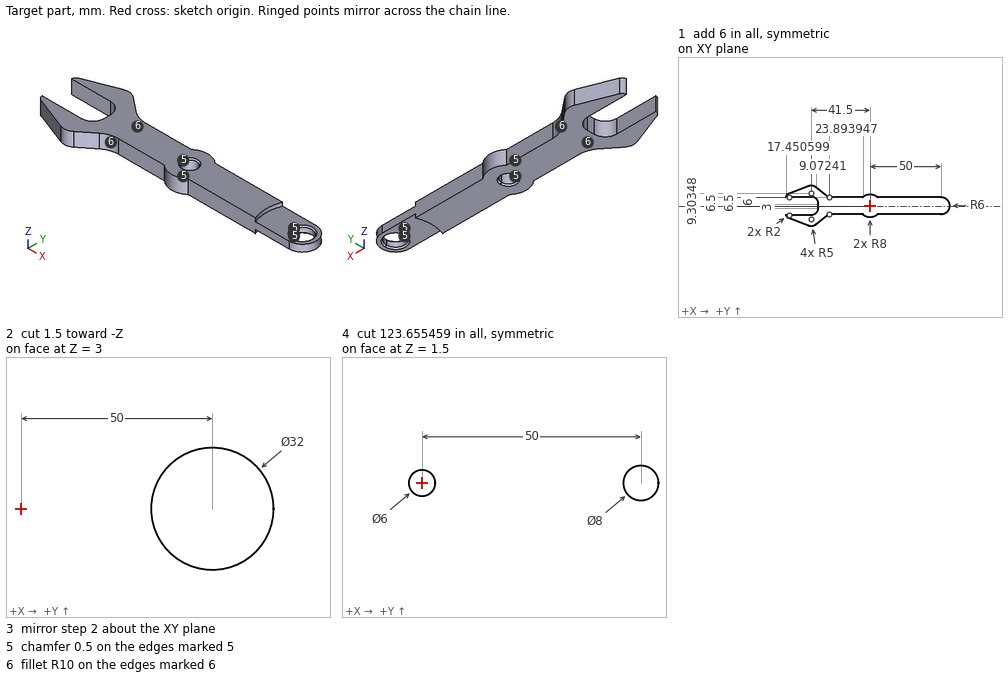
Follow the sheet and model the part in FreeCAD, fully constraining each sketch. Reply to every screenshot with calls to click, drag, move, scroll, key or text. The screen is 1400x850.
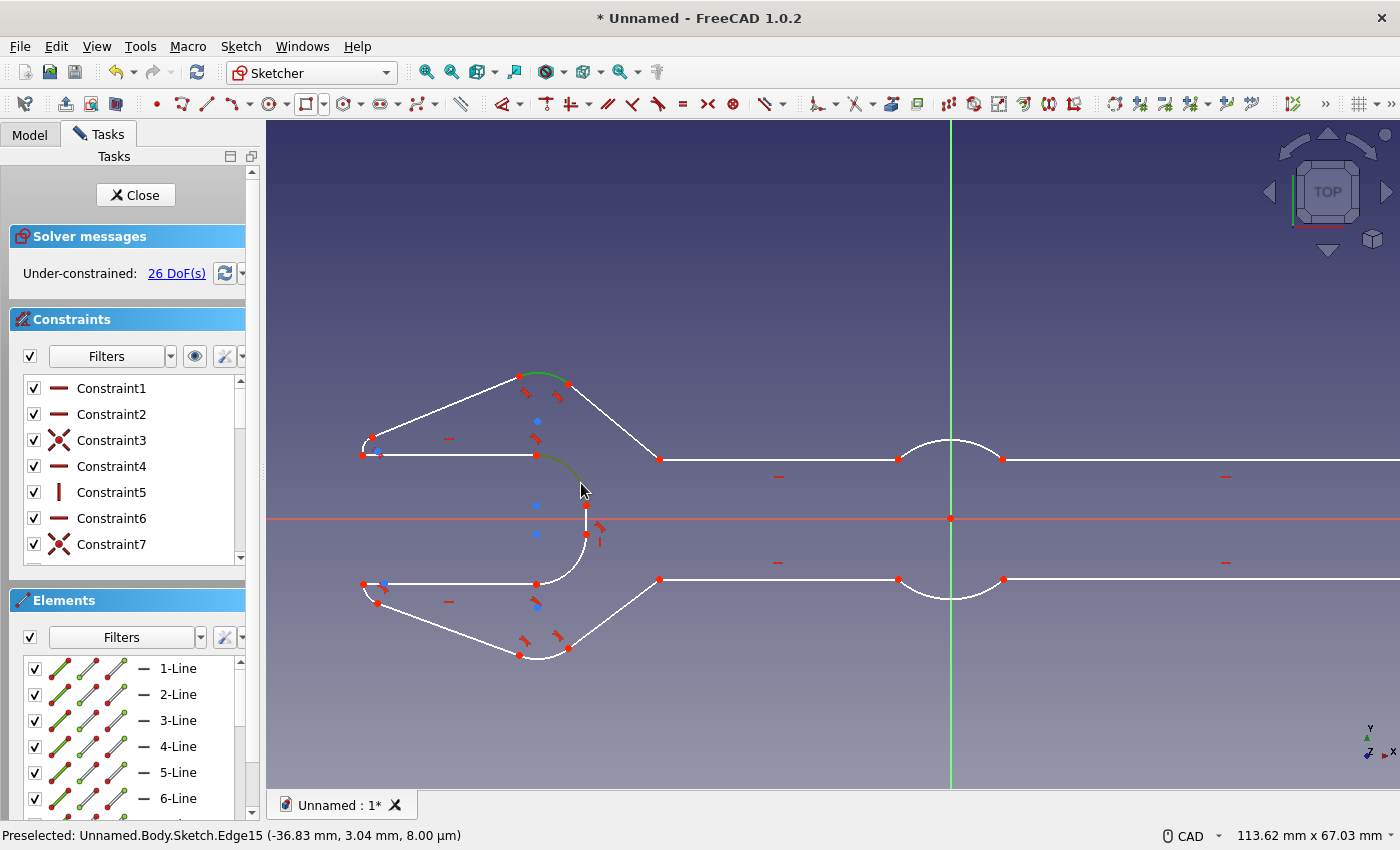
click(559, 579)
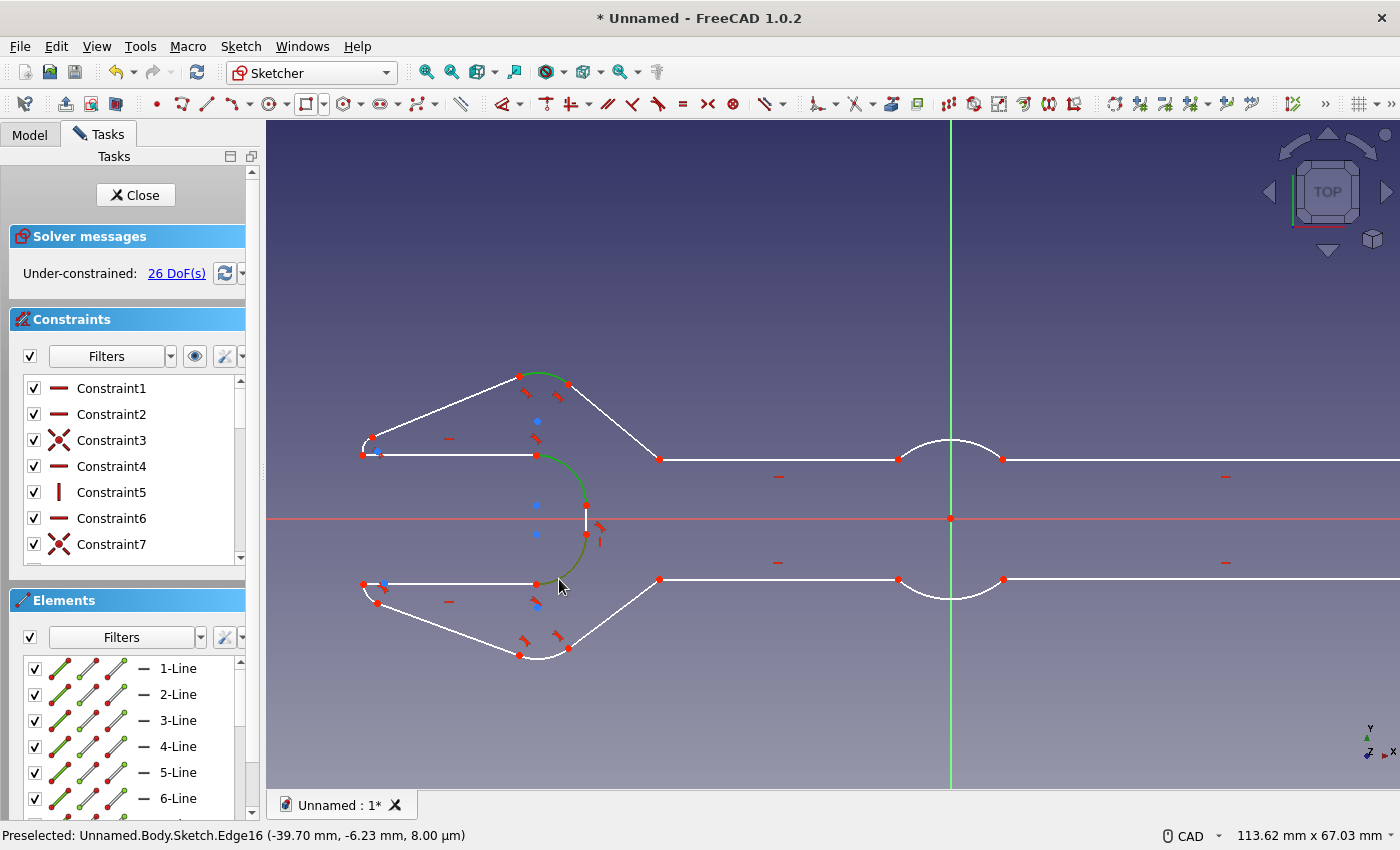
click(535, 659)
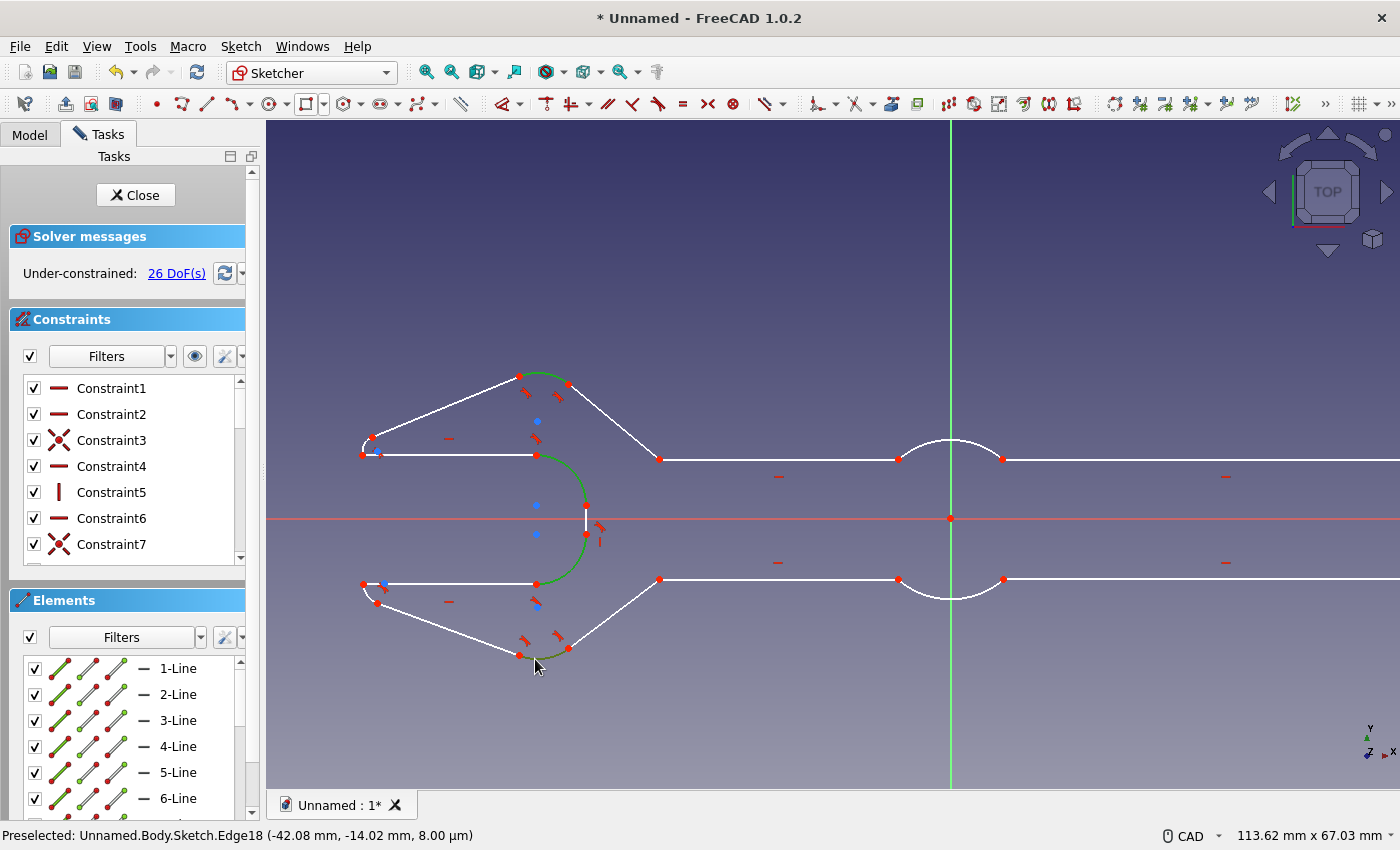
click(683, 104)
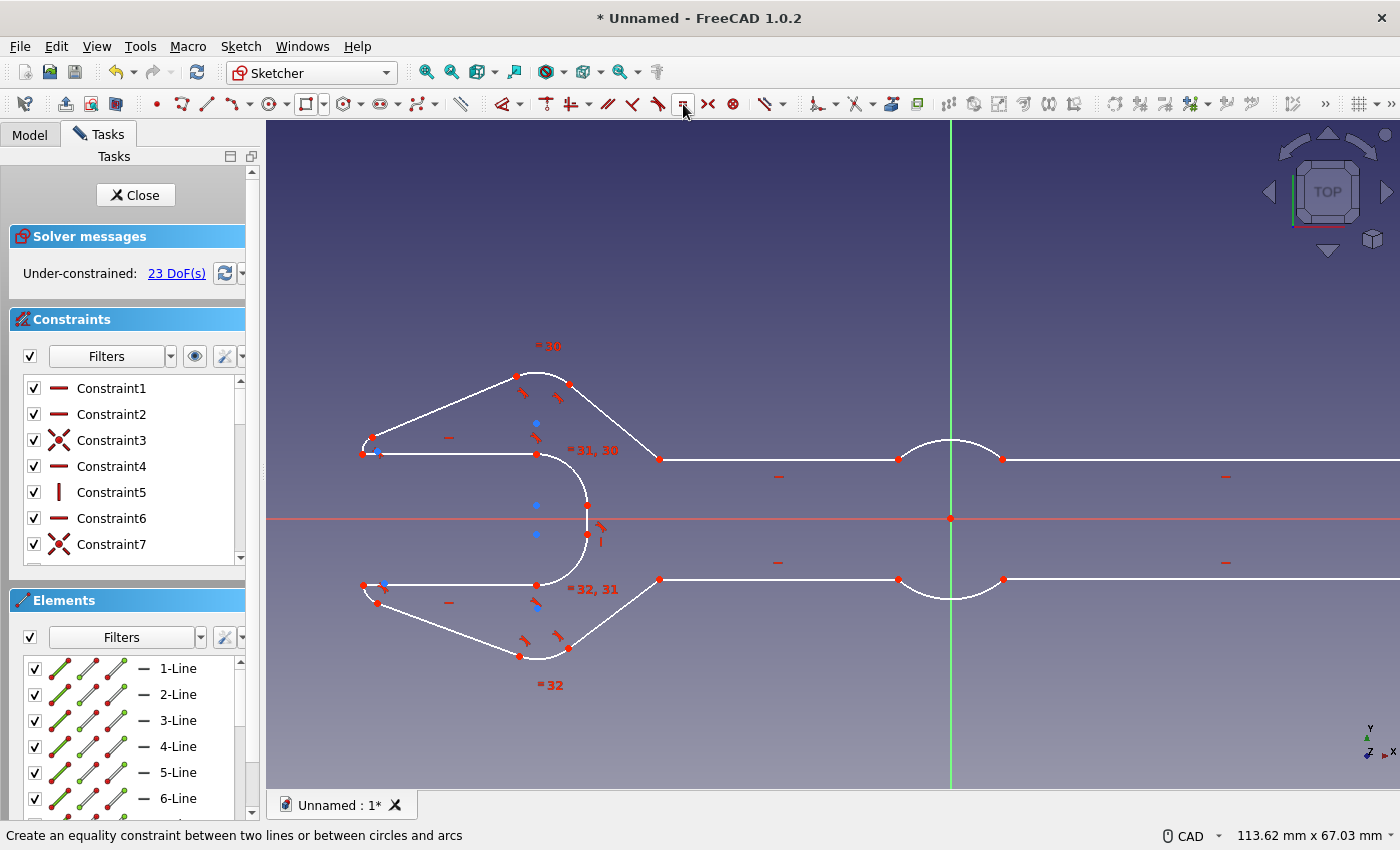
scroll(365, 444, up, 2)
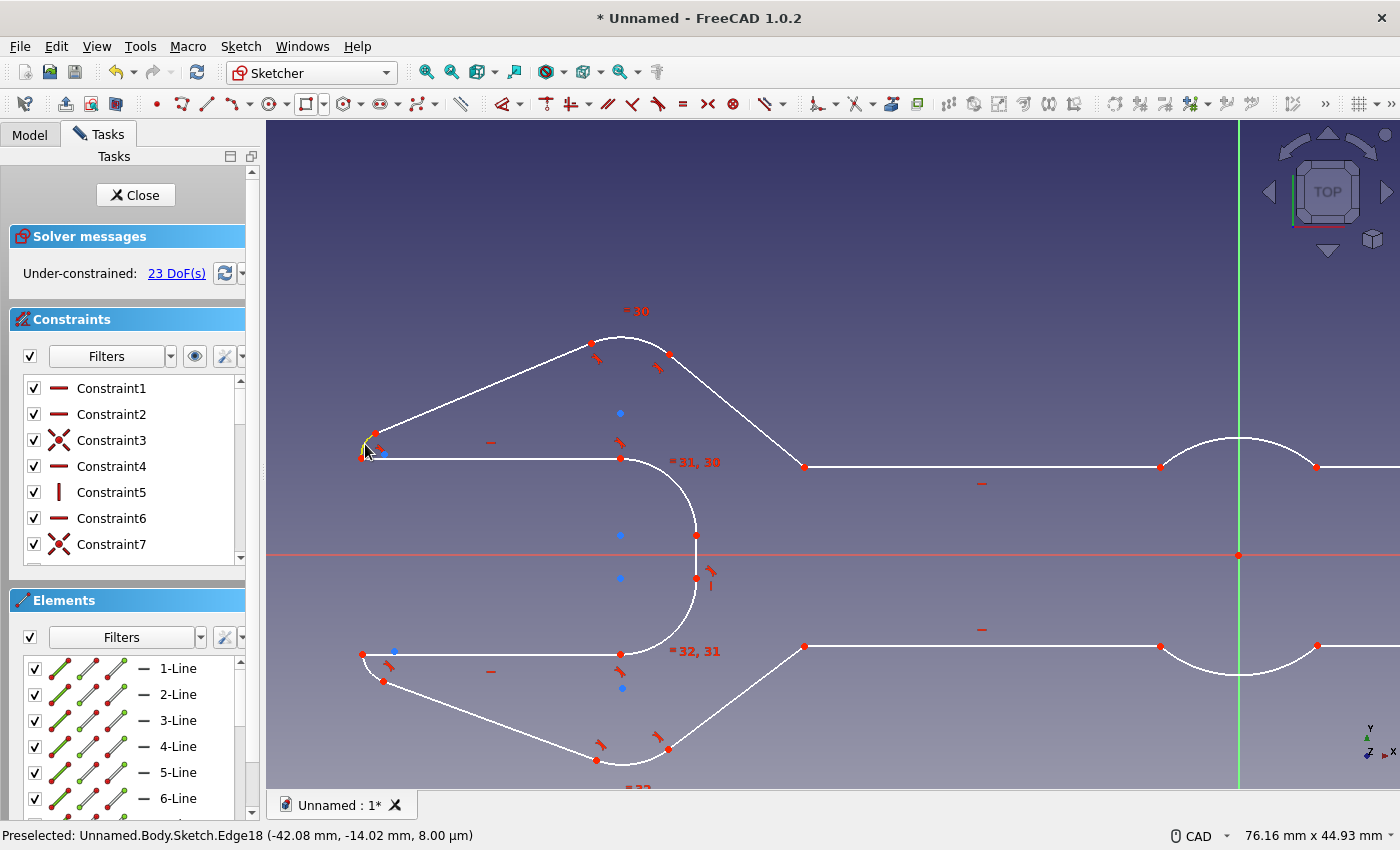
click(364, 444)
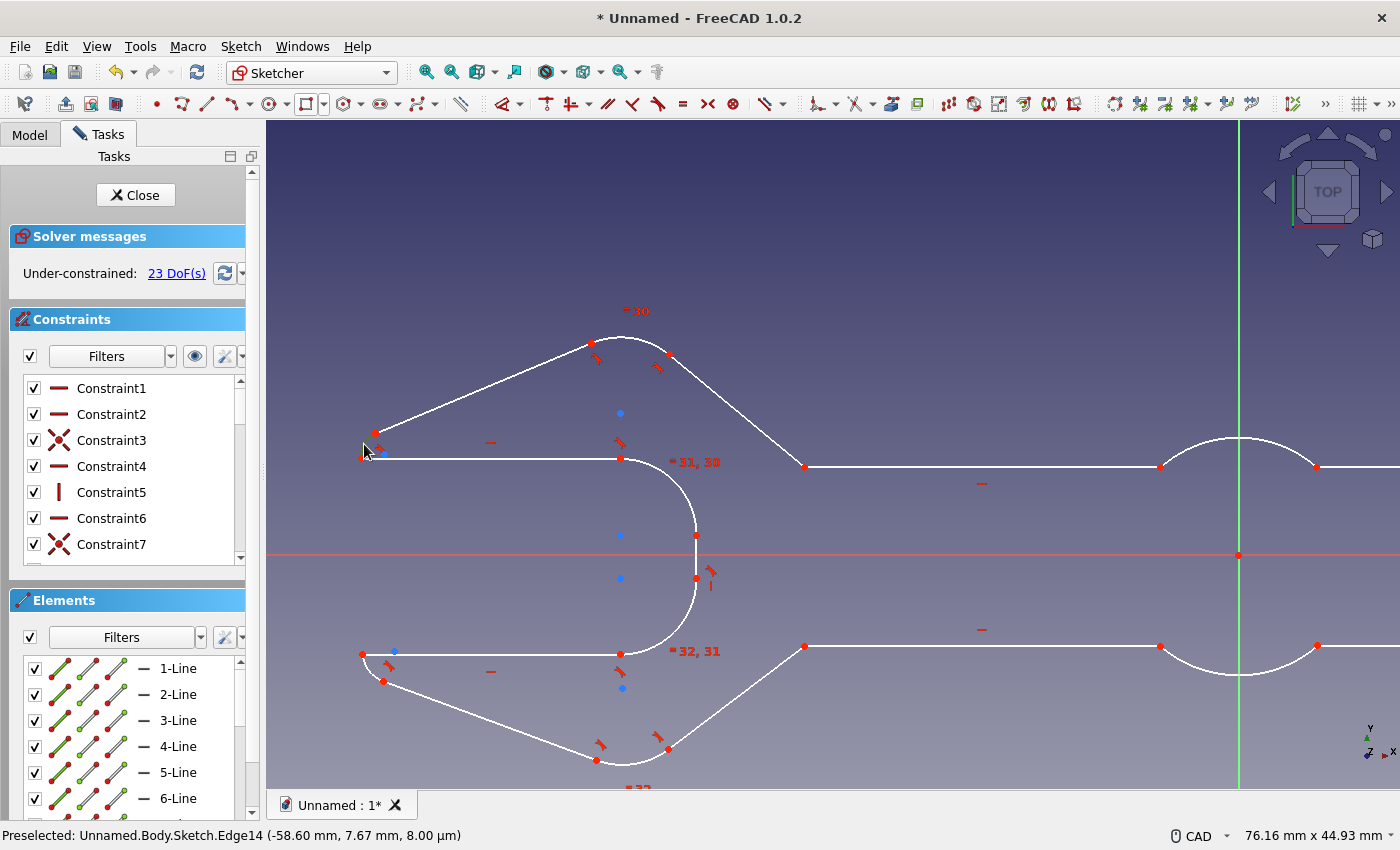
scroll(365, 665, up, 2)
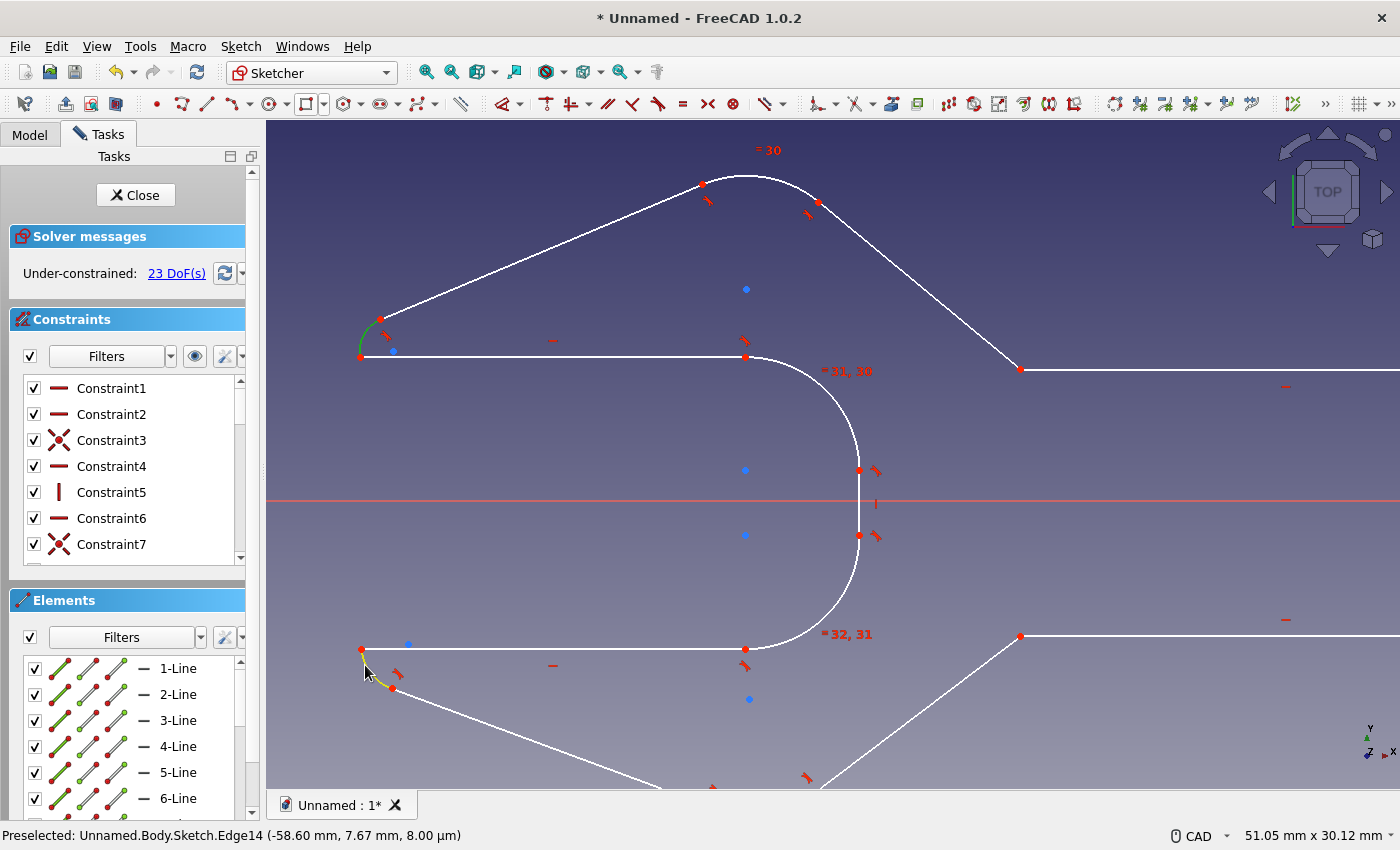
click(366, 664)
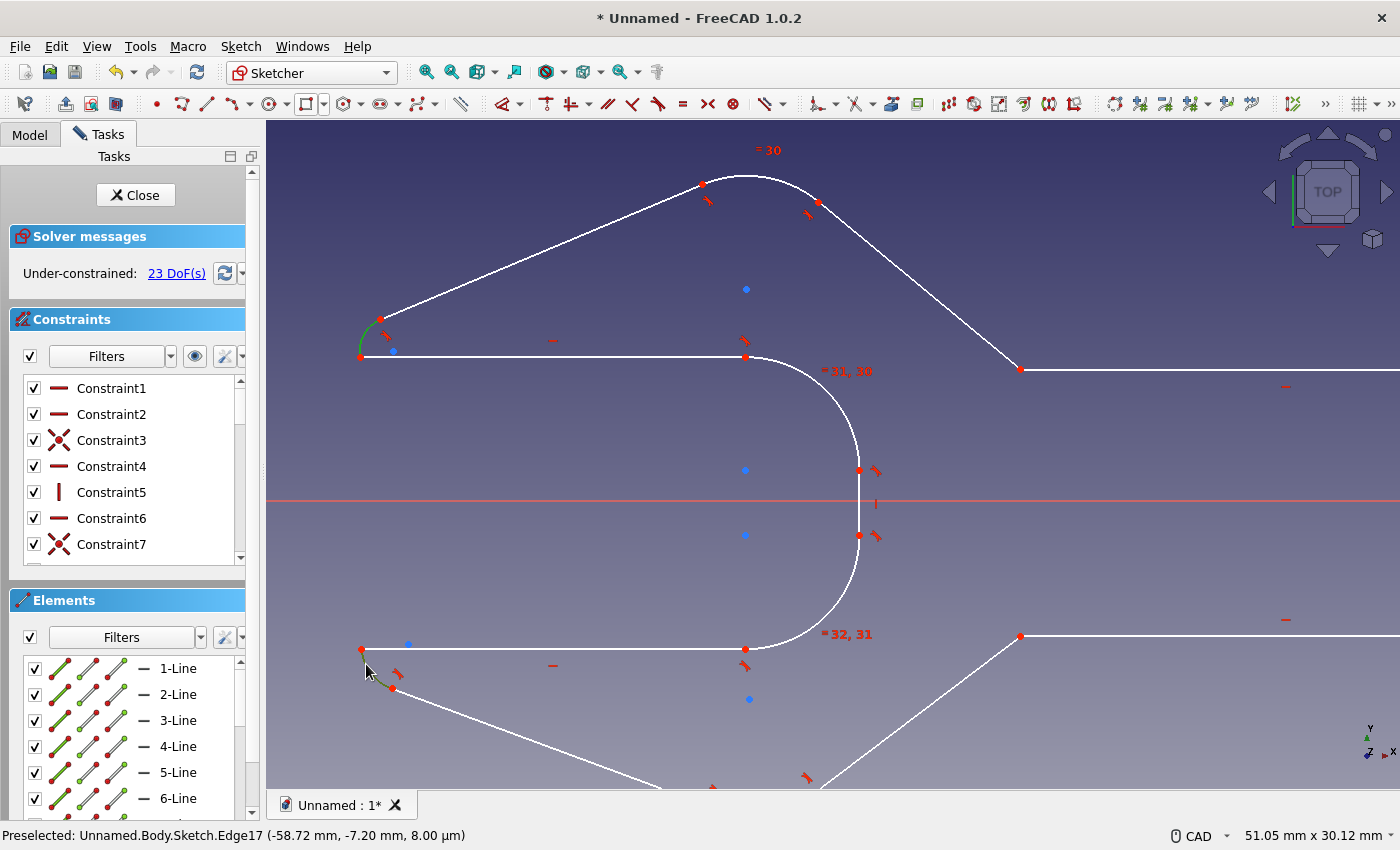
click(683, 104)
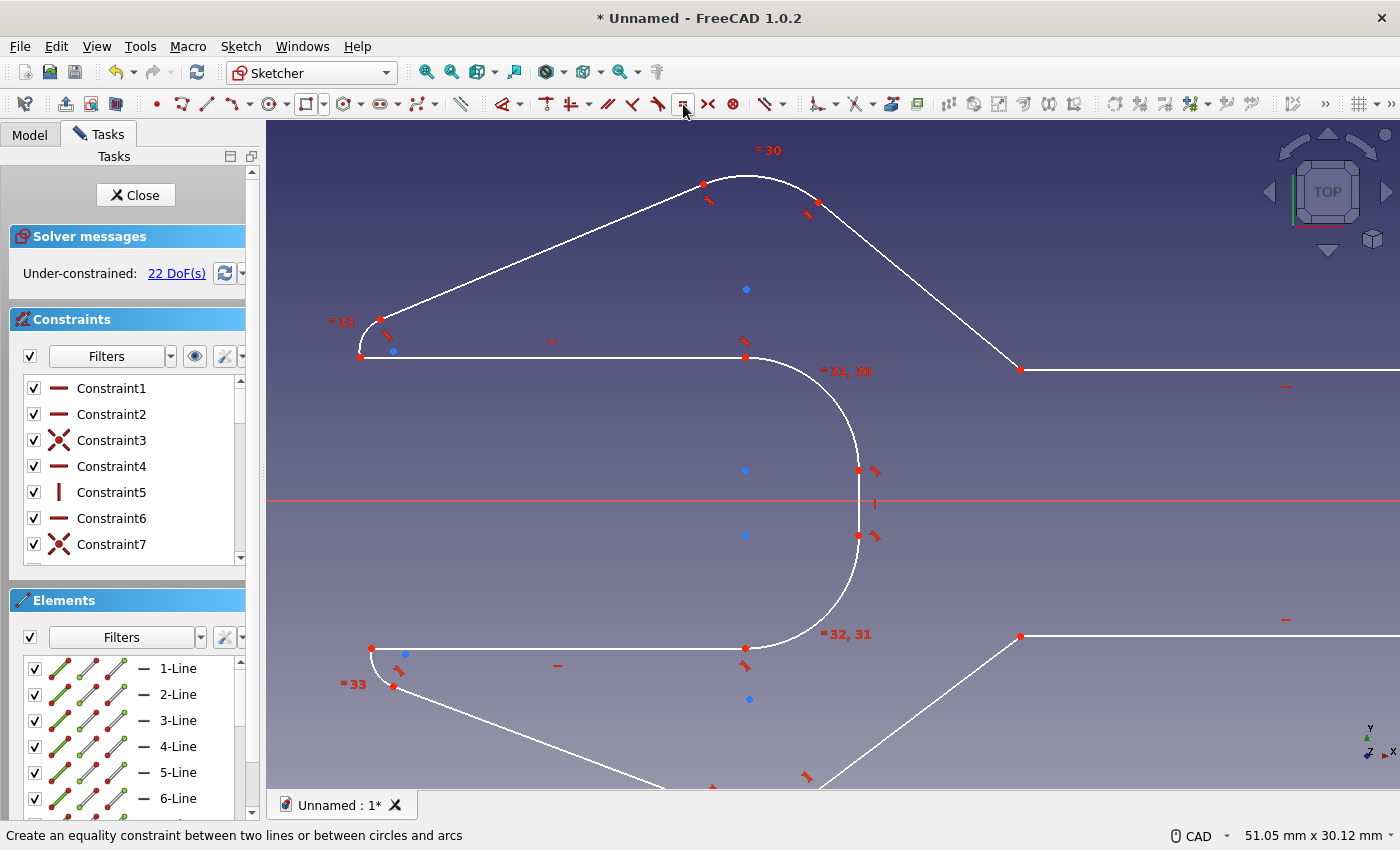
scroll(479, 439, down, 7)